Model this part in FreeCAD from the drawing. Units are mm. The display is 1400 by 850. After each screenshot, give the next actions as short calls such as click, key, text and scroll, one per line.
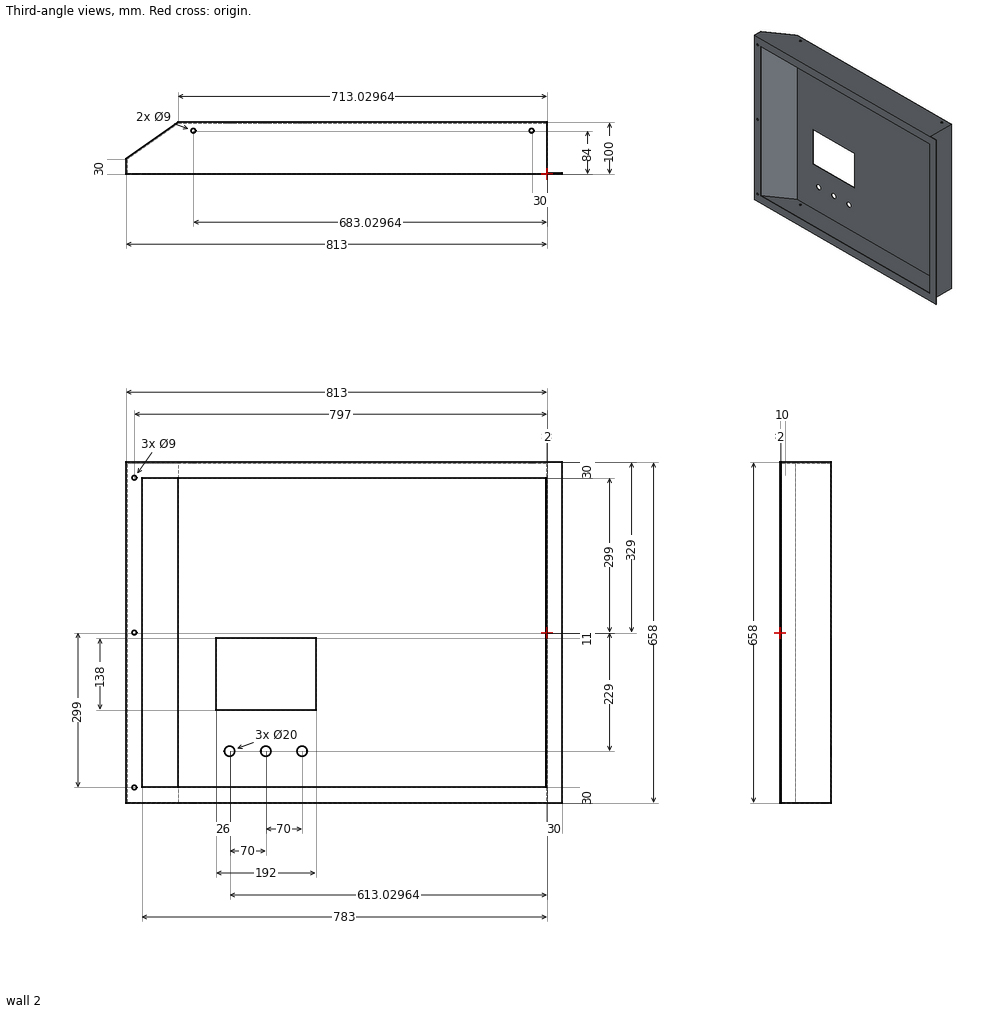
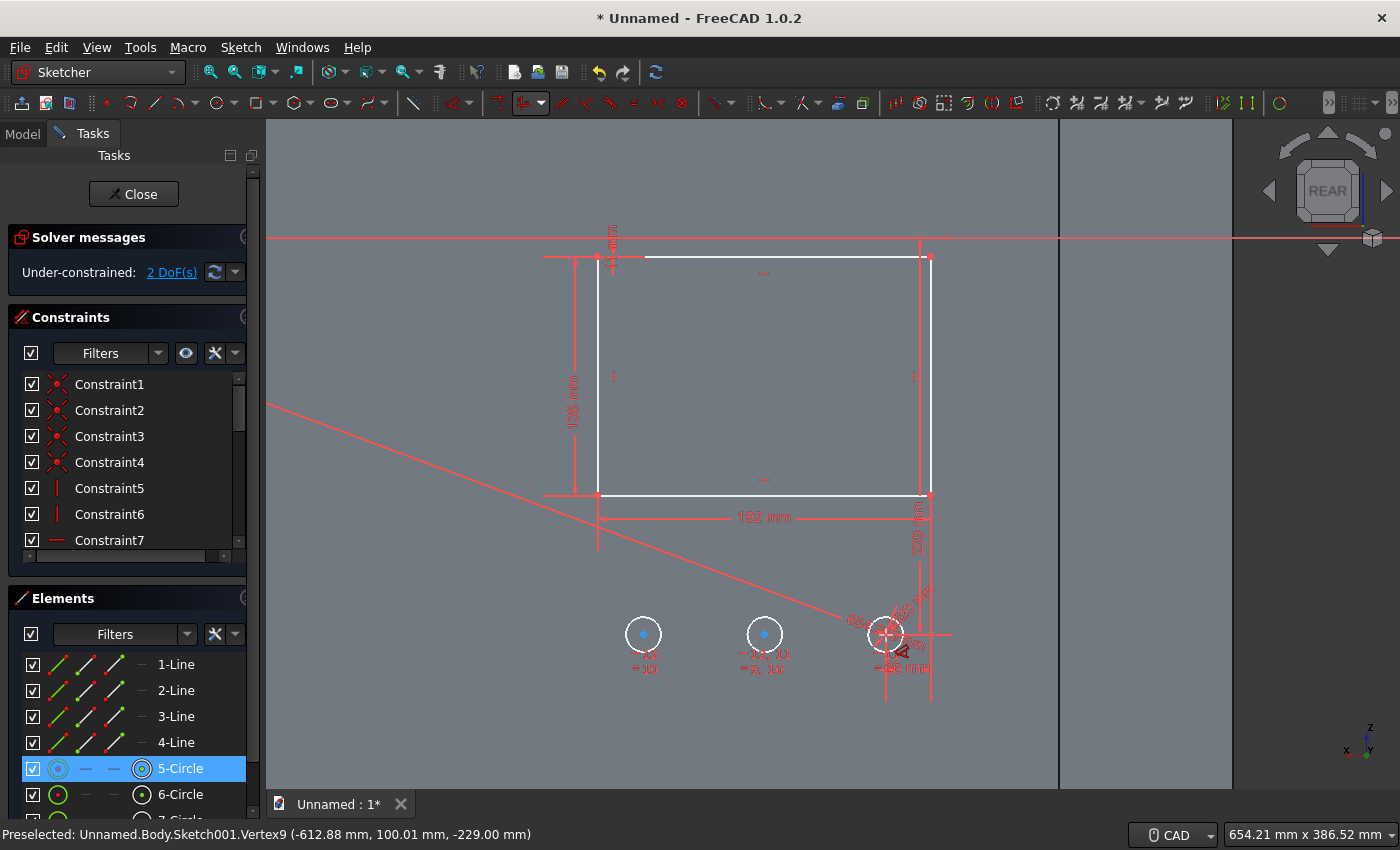
click(765, 635)
click(825, 669)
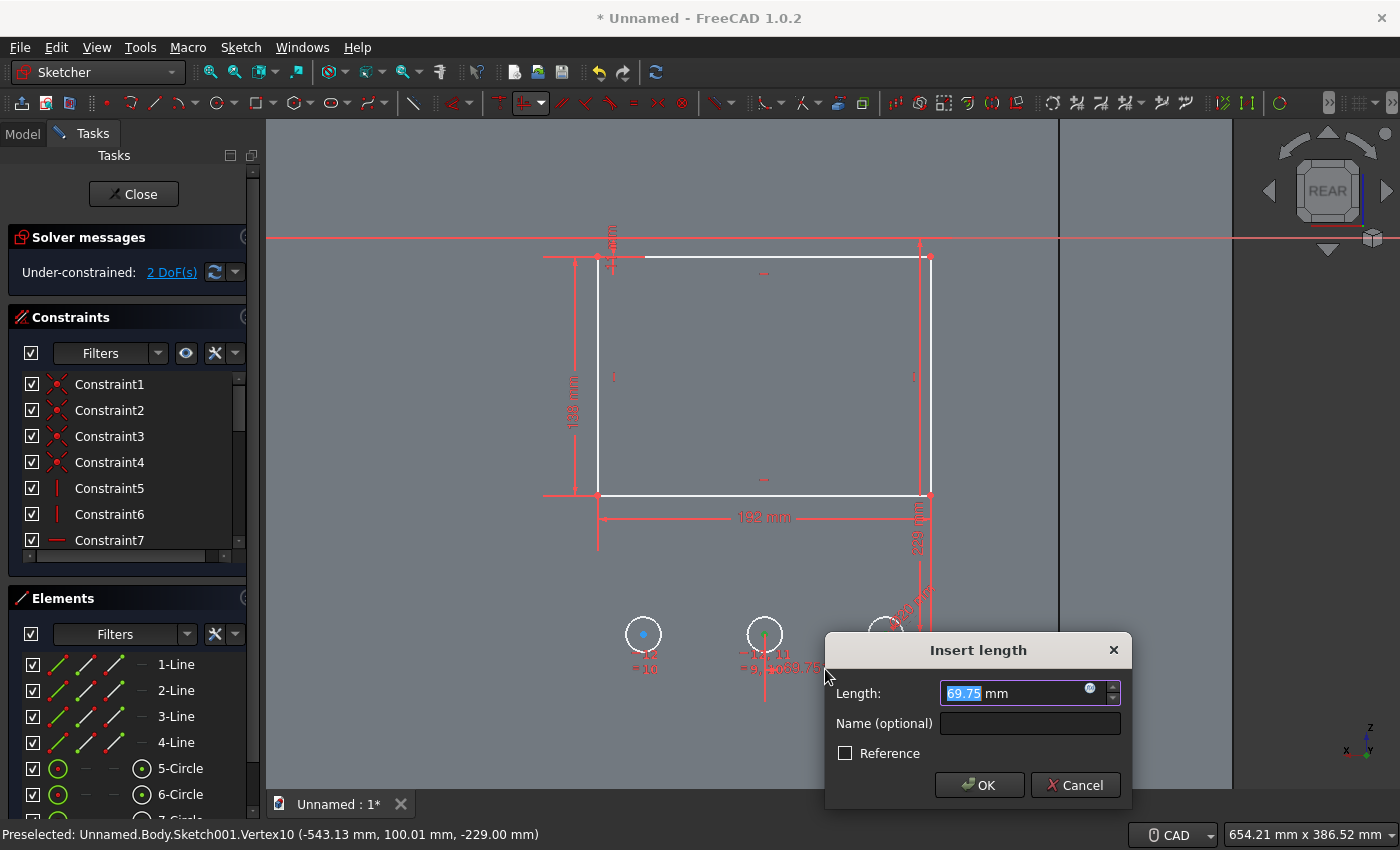
text(70)
key(Return)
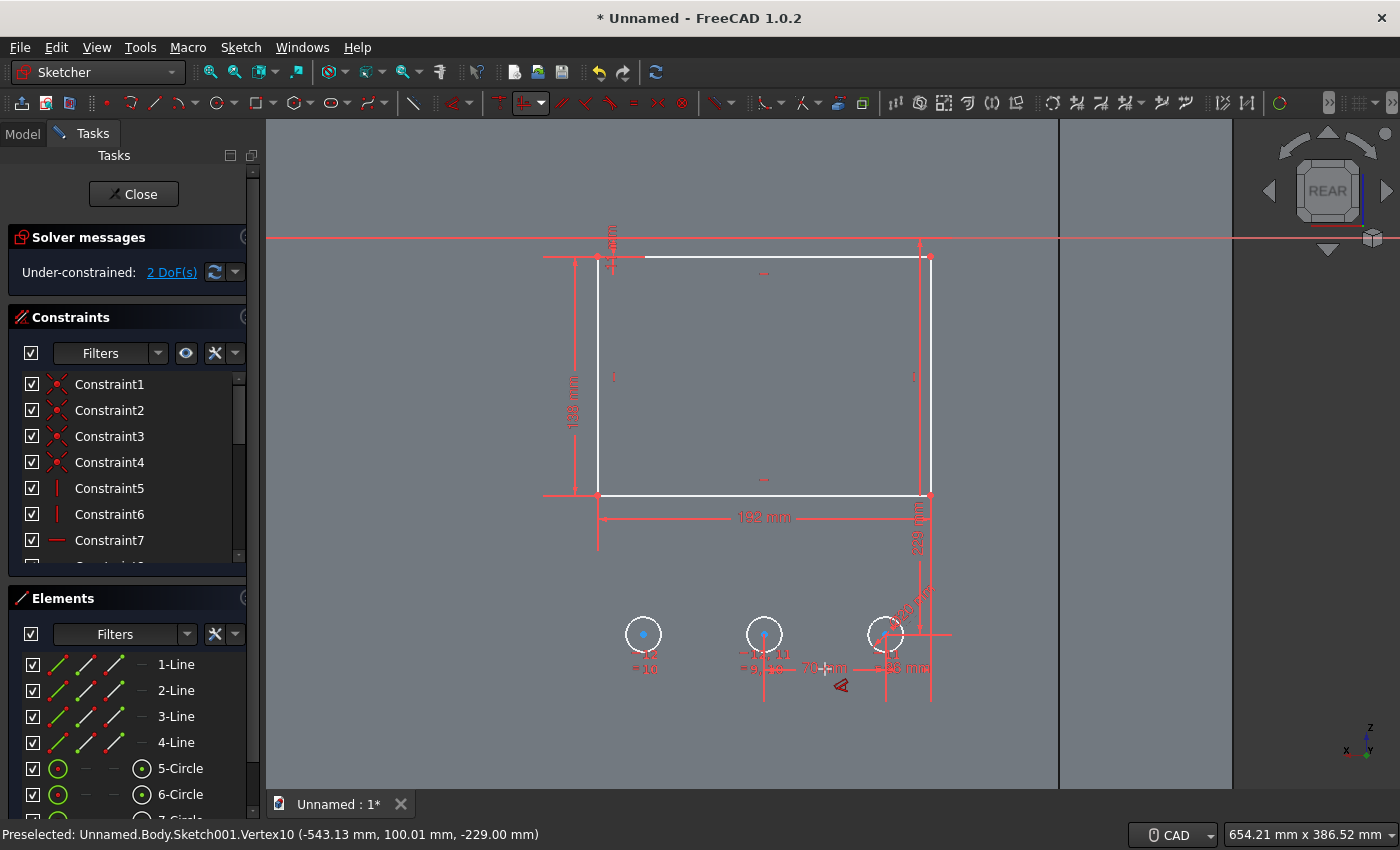
click(764, 635)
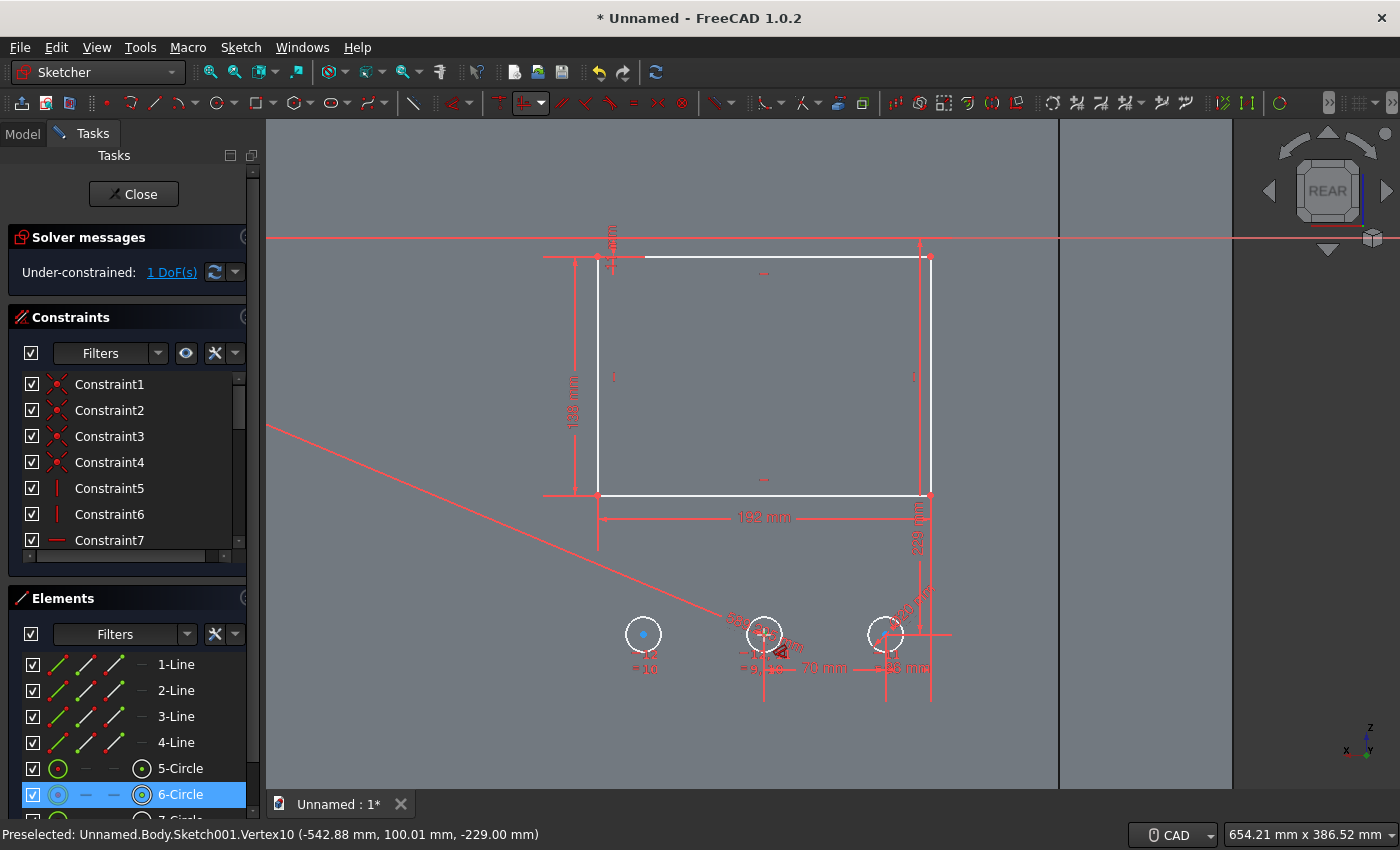
click(644, 635)
click(704, 669)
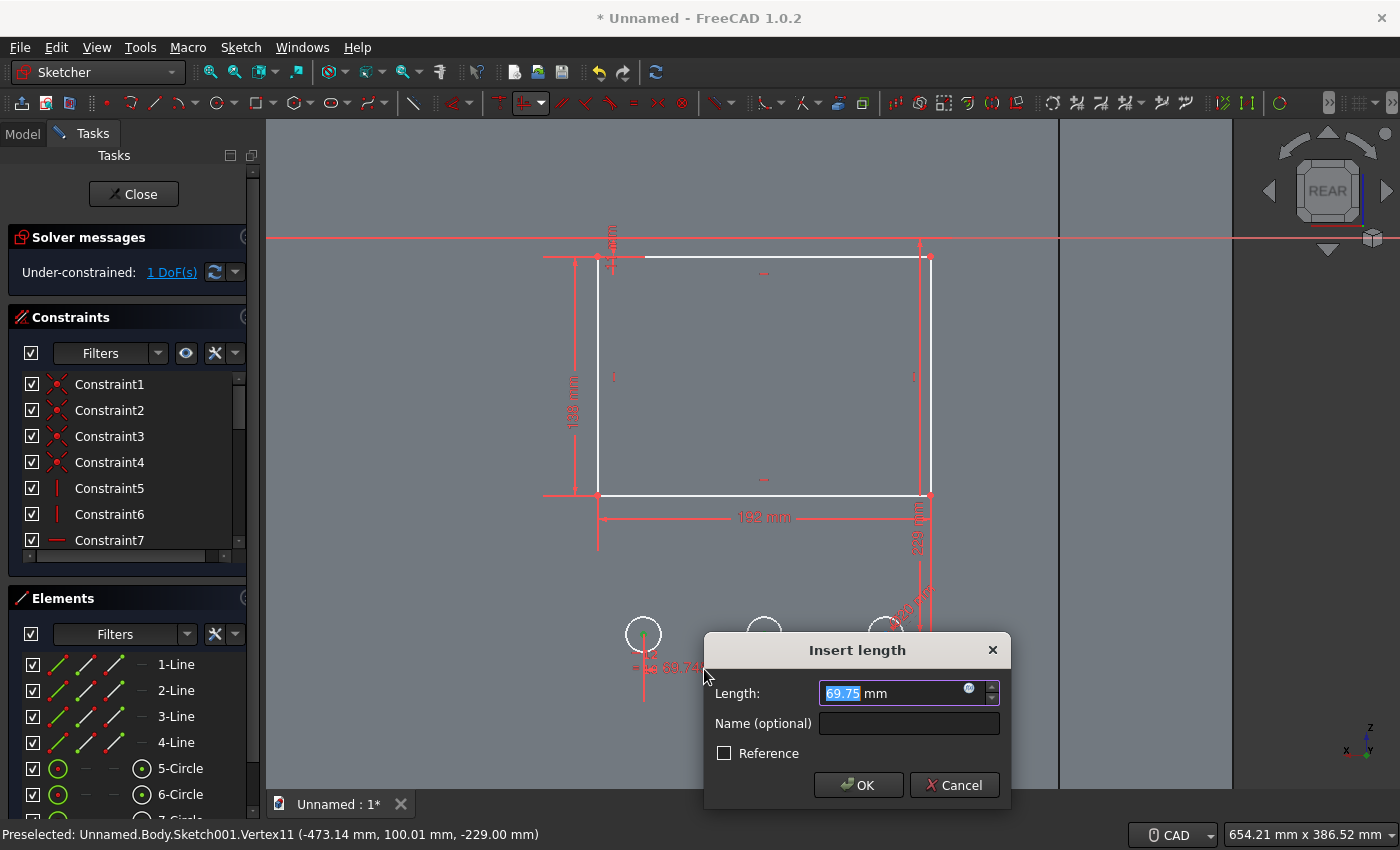
text(70)
key(Return)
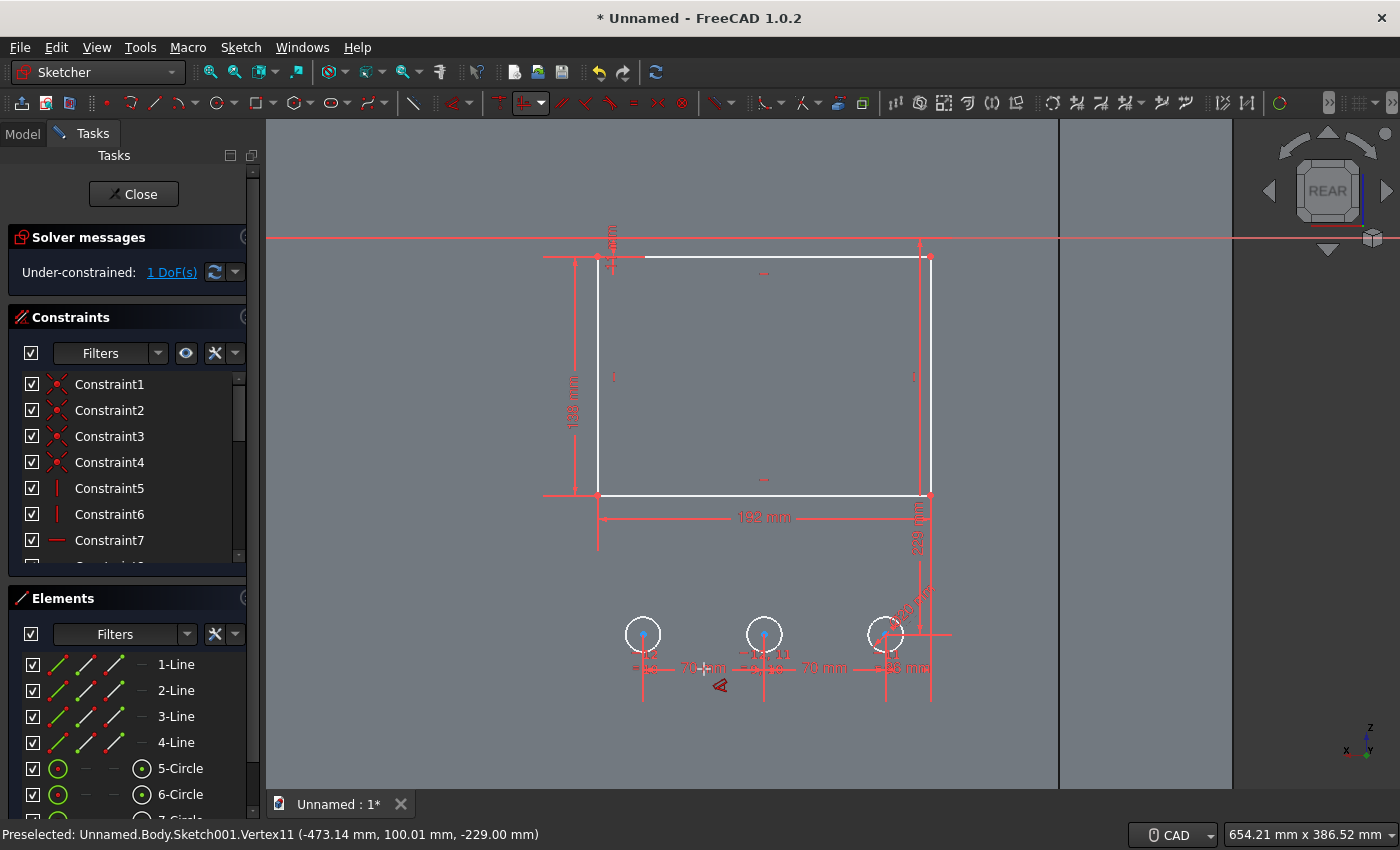
click(886, 635)
click(590, 204)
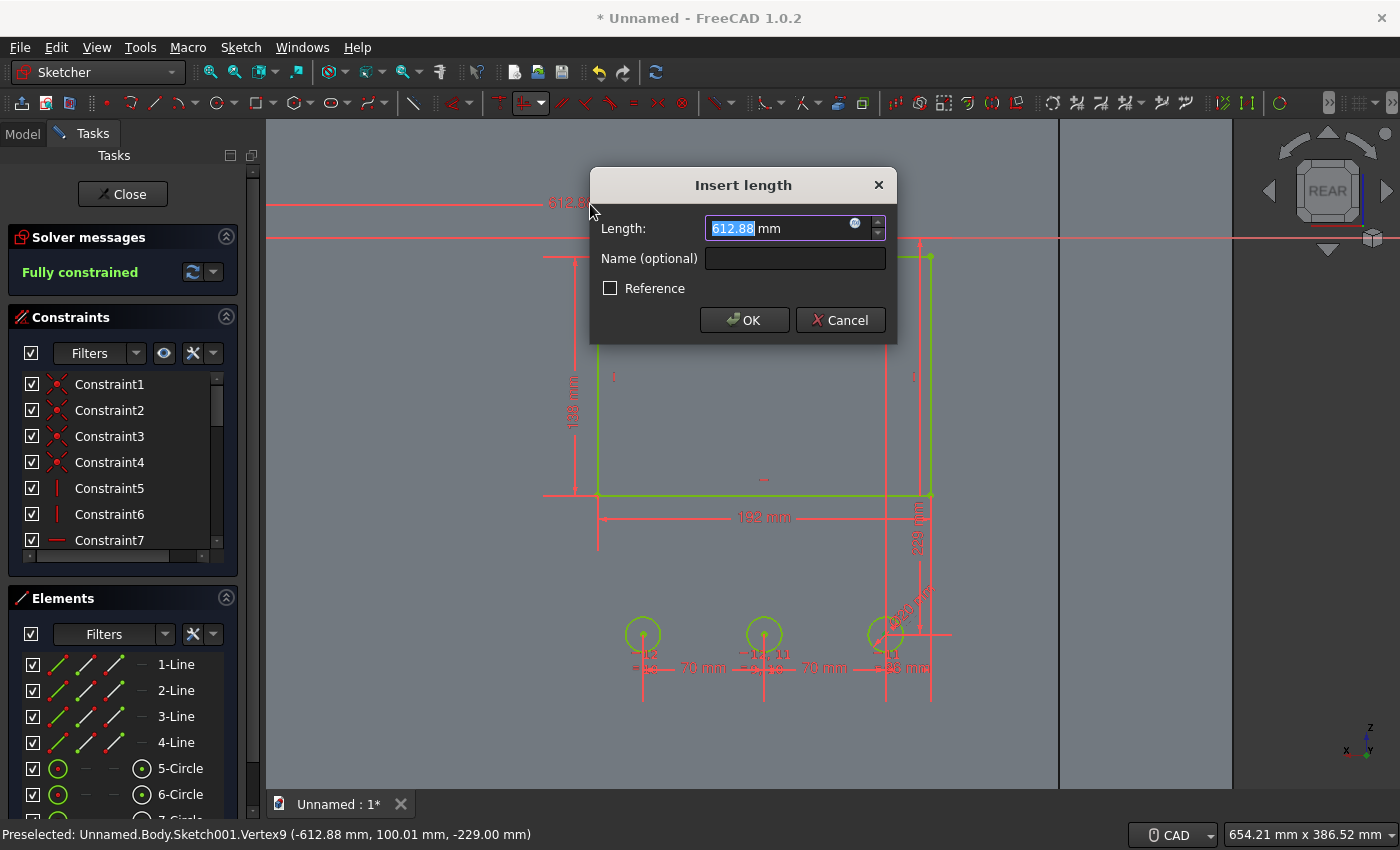
text(613.02964)
key(Return)
key(Escape)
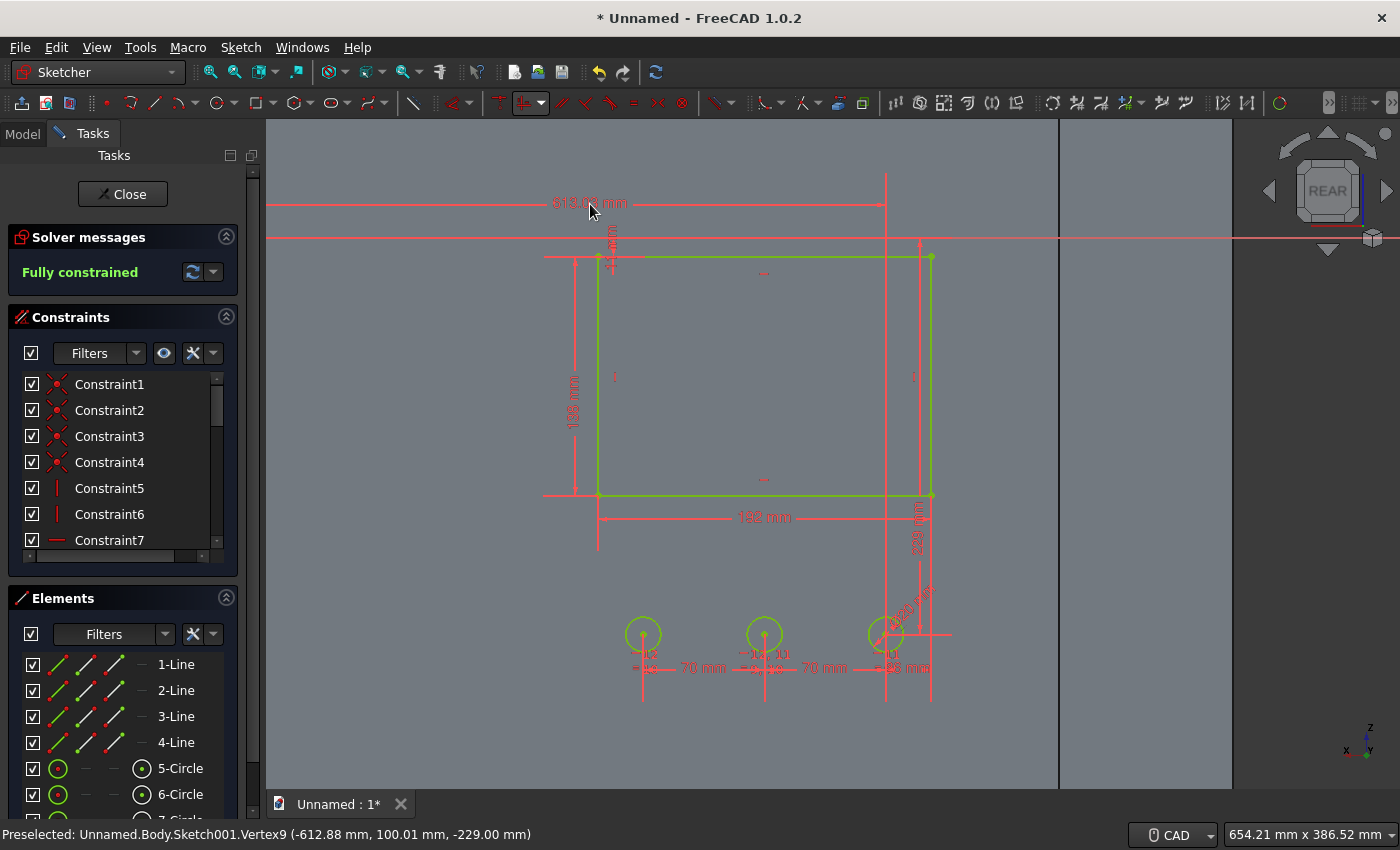
click(123, 194)